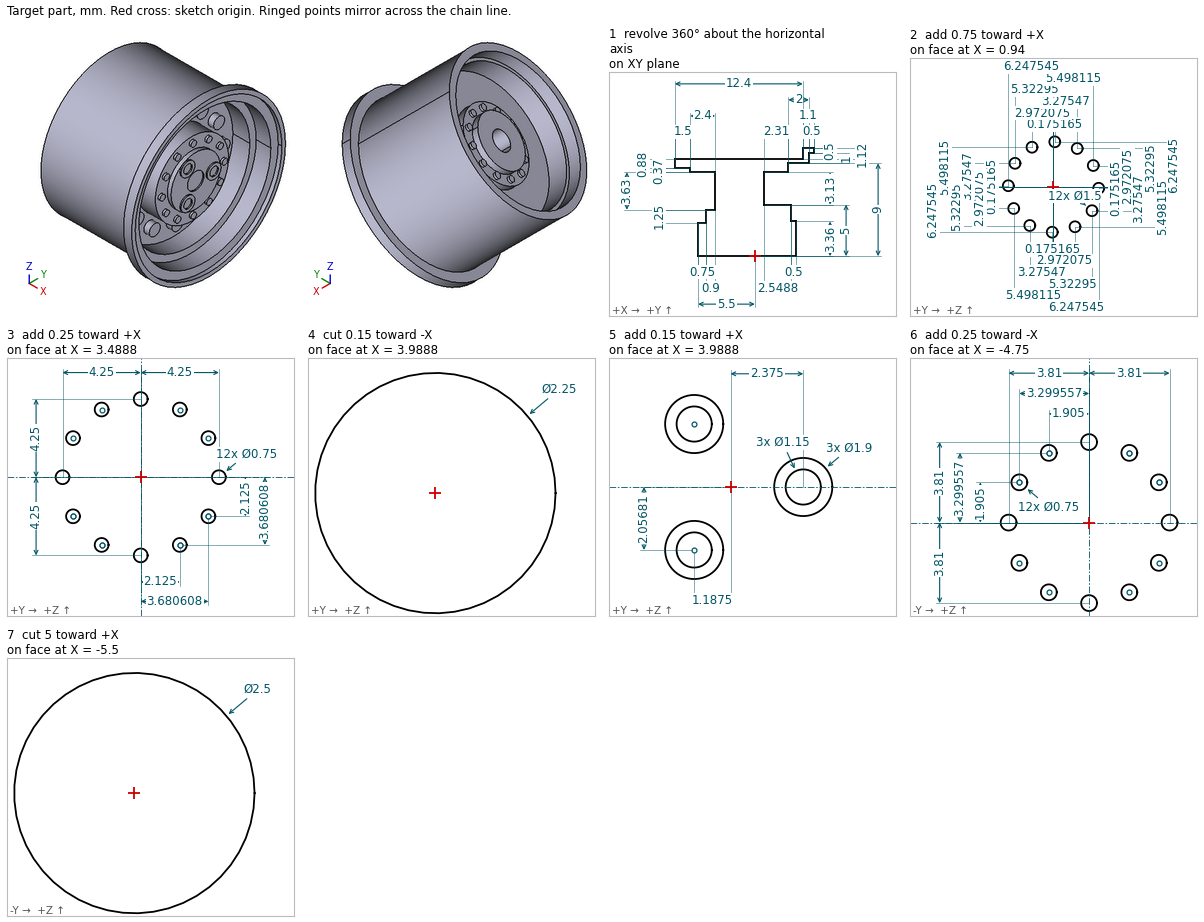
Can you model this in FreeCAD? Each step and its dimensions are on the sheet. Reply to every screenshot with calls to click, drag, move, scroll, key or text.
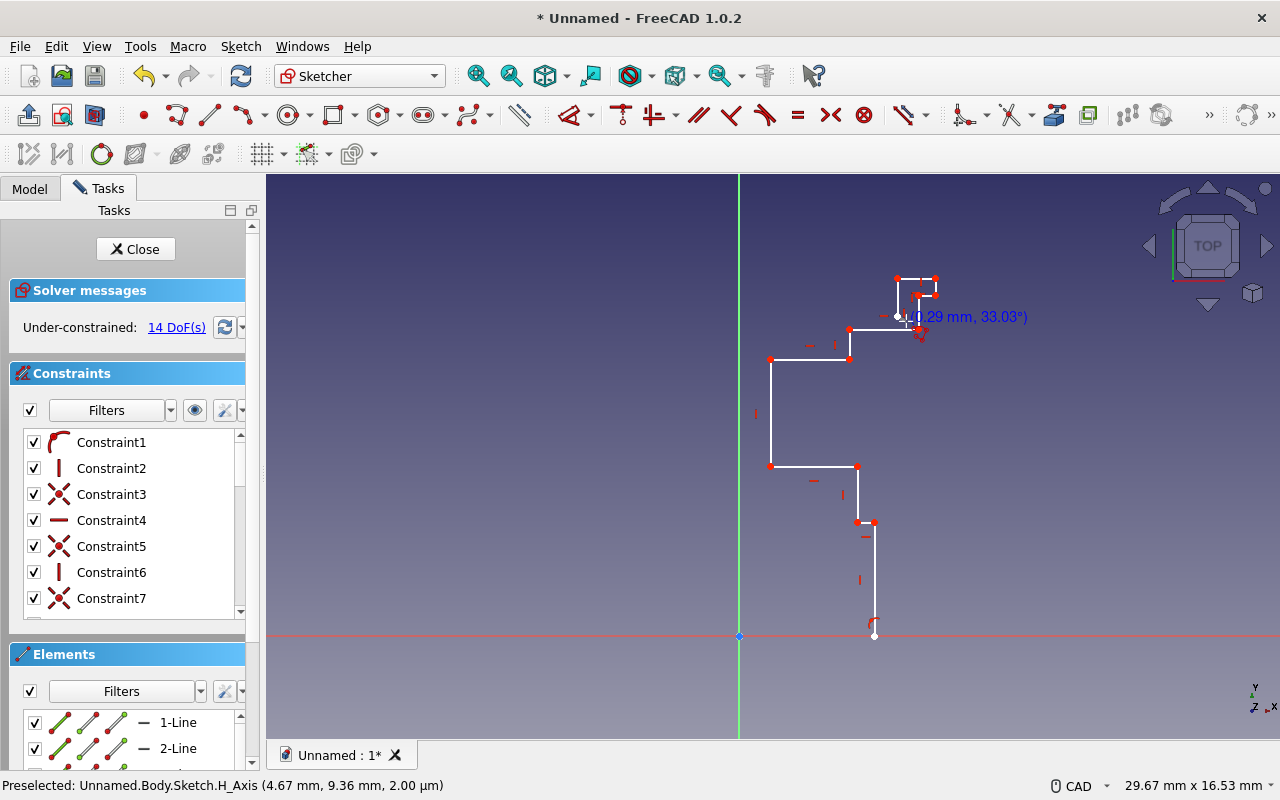
click(474, 316)
click(474, 346)
click(525, 346)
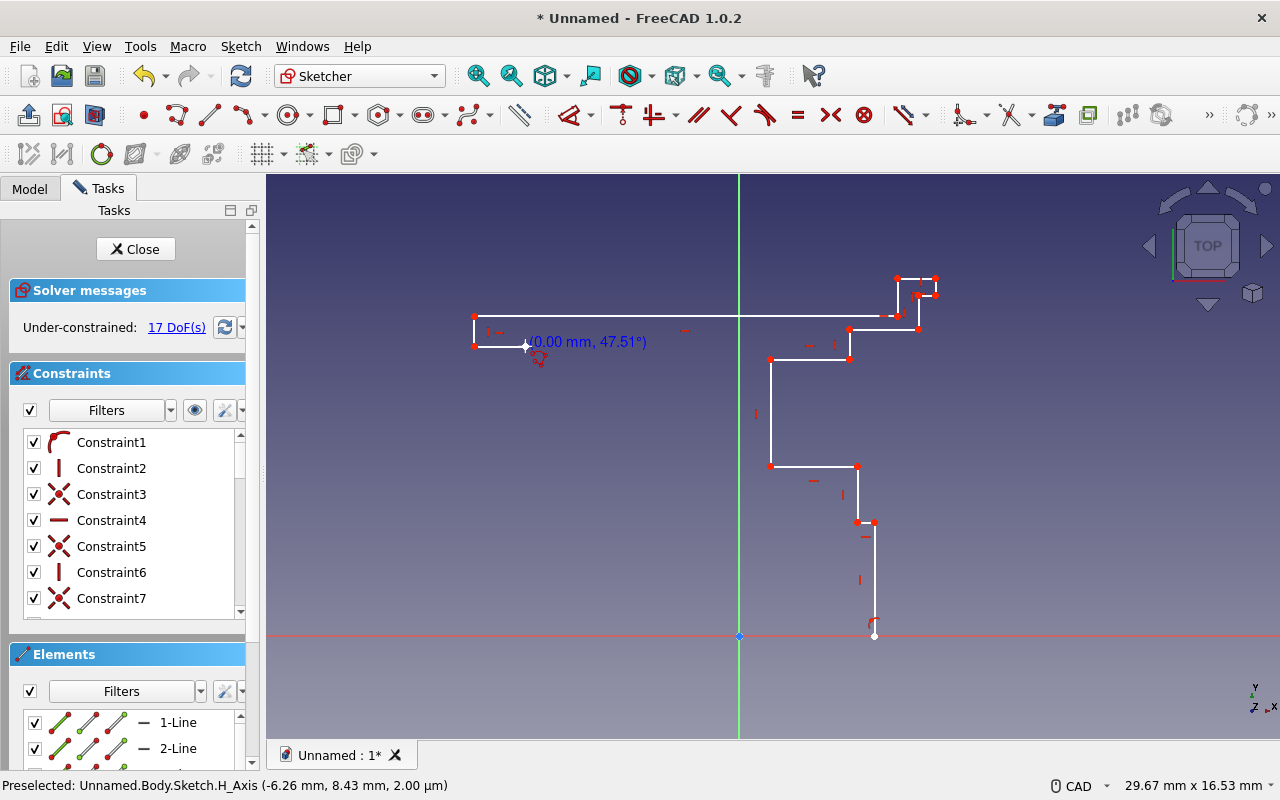
scroll(525, 358, up, 2)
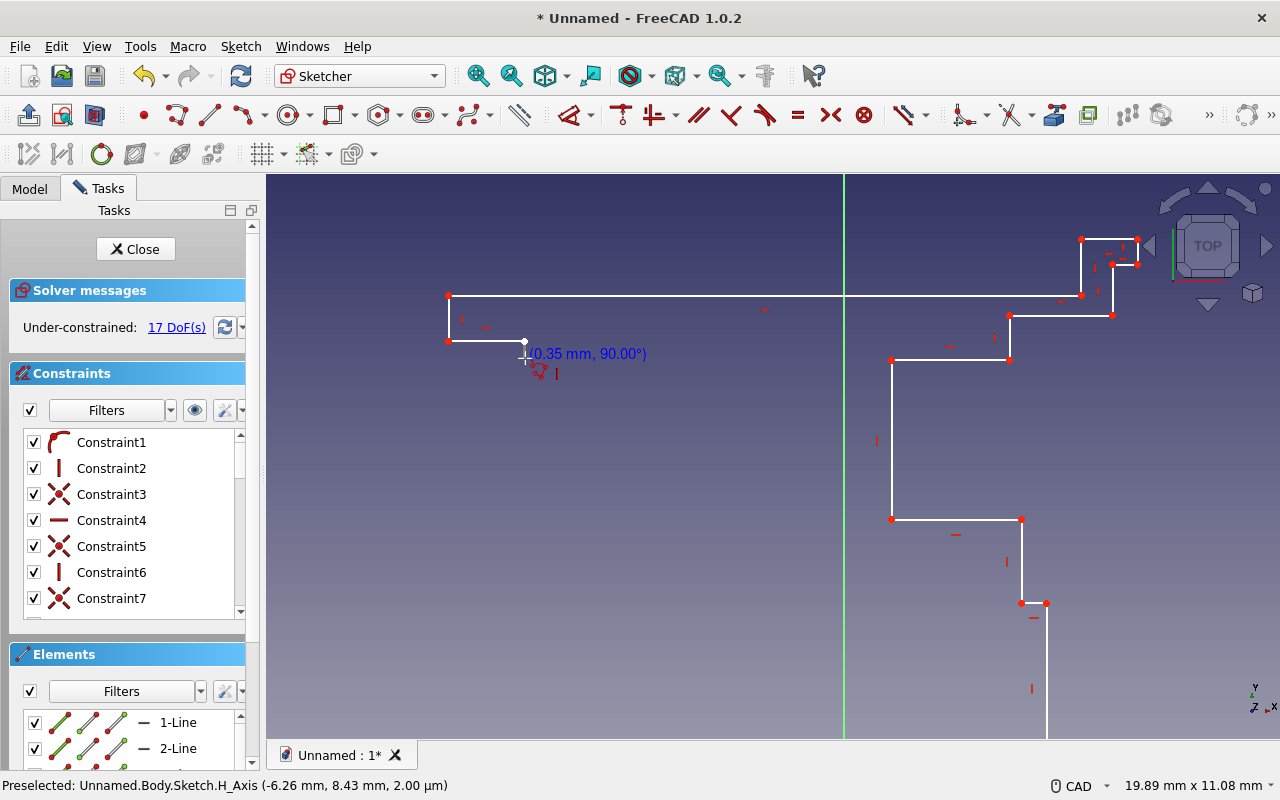
click(525, 358)
click(648, 358)
click(648, 543)
click(602, 543)
click(602, 607)
click(564, 607)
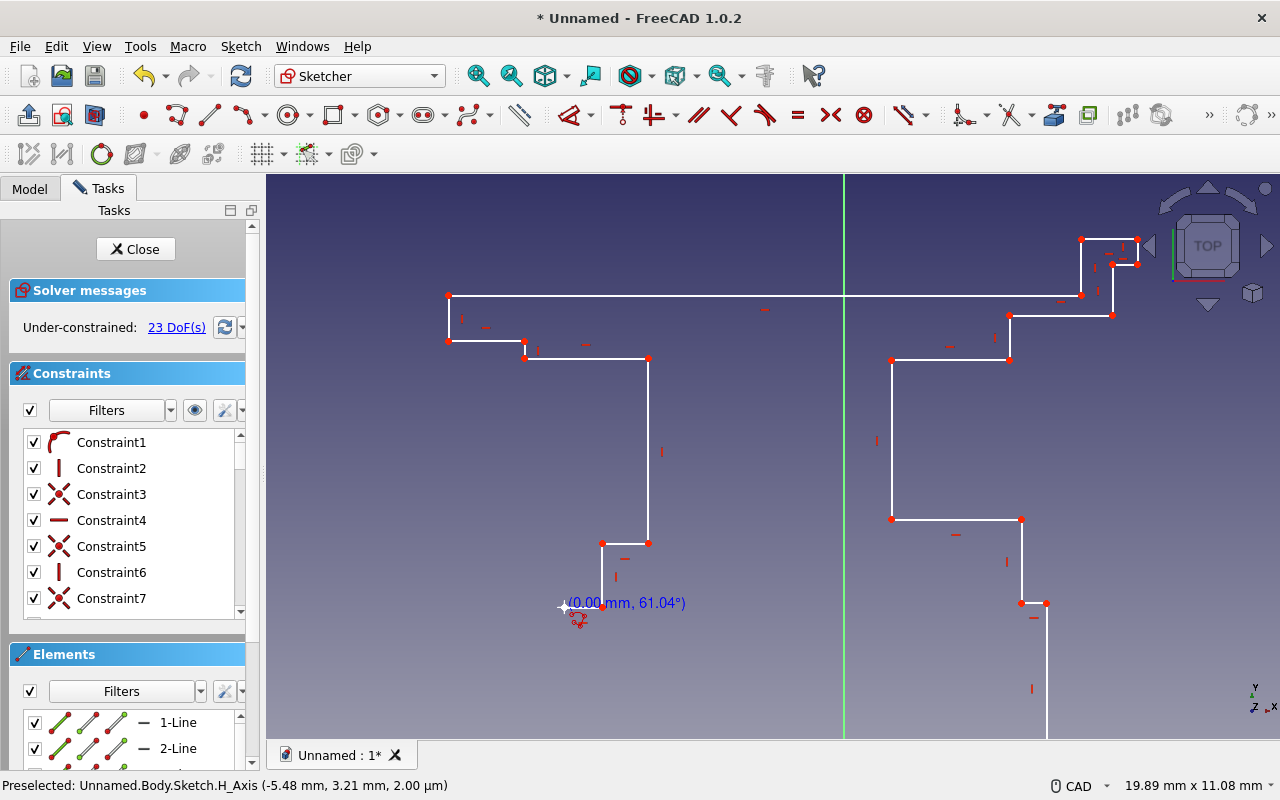
scroll(524, 358, down, 2)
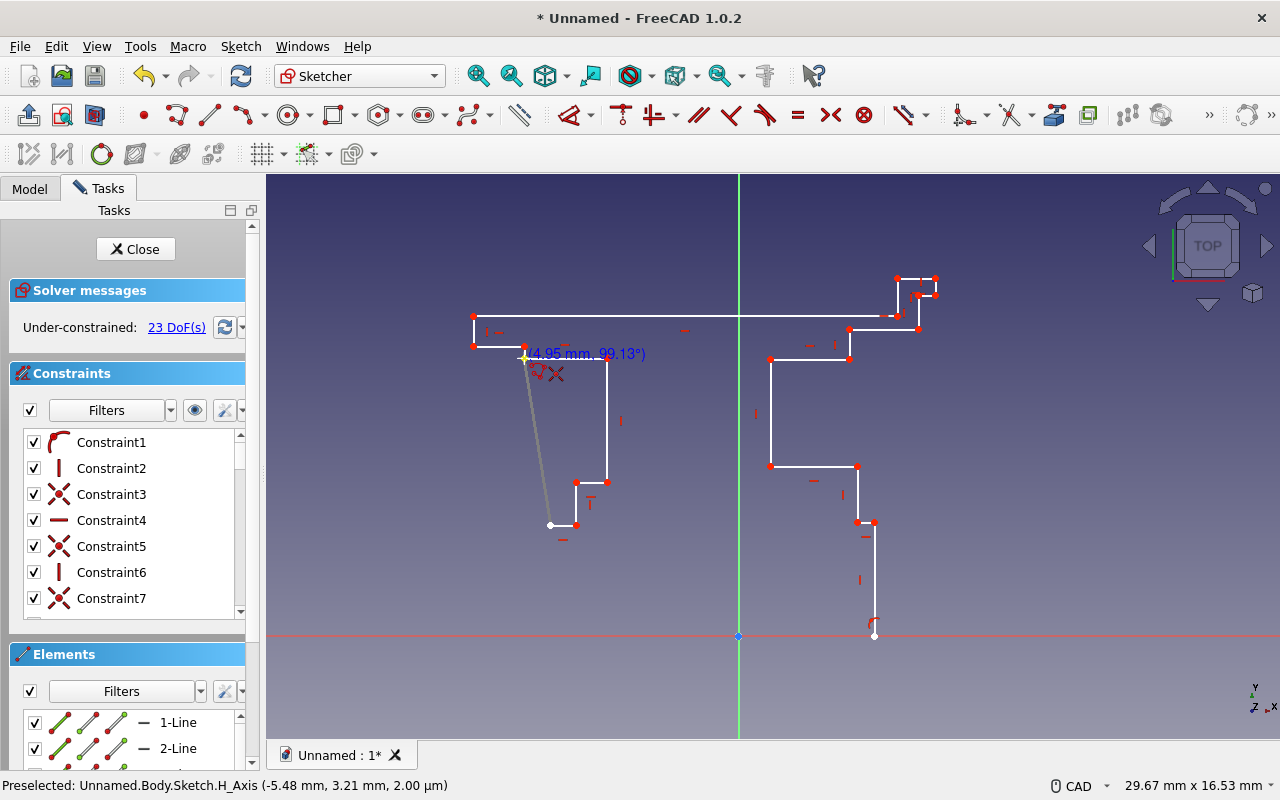
click(551, 627)
click(875, 636)
key(Escape)
key(Escape)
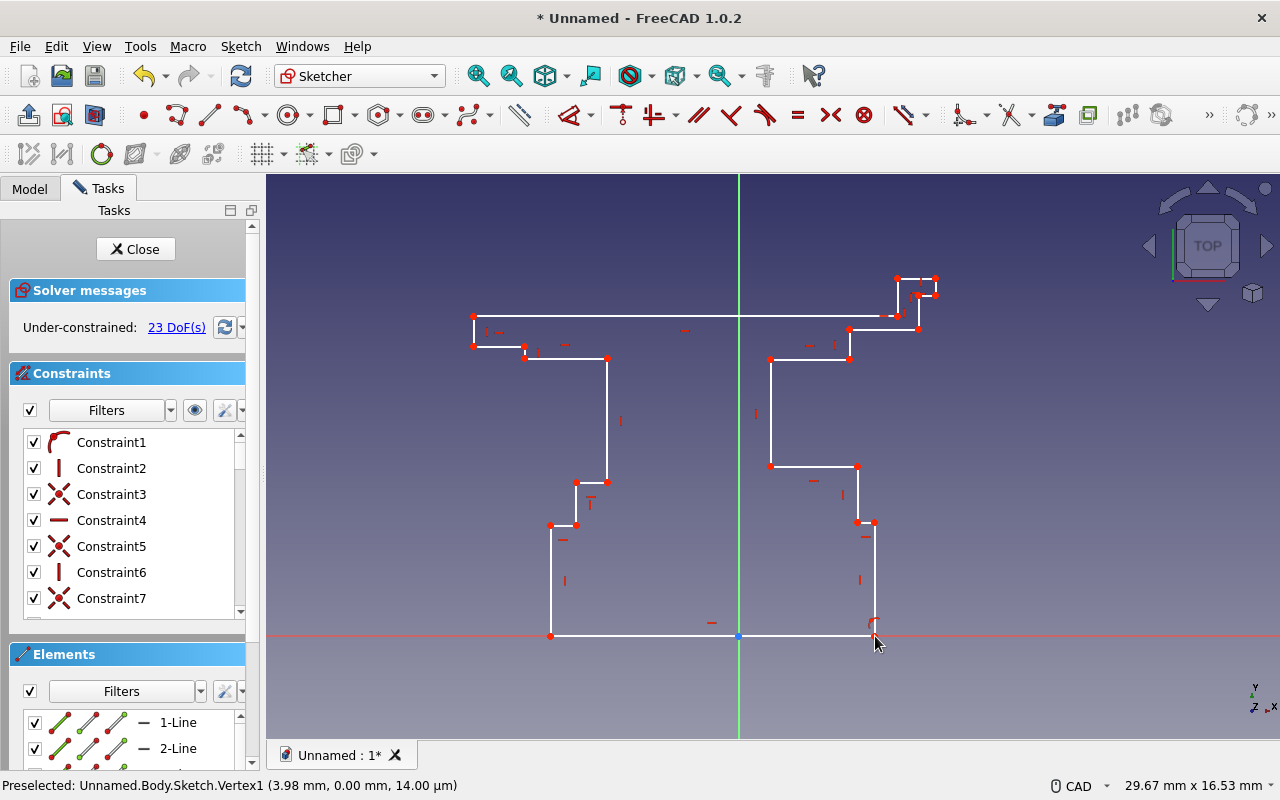
click(568, 116)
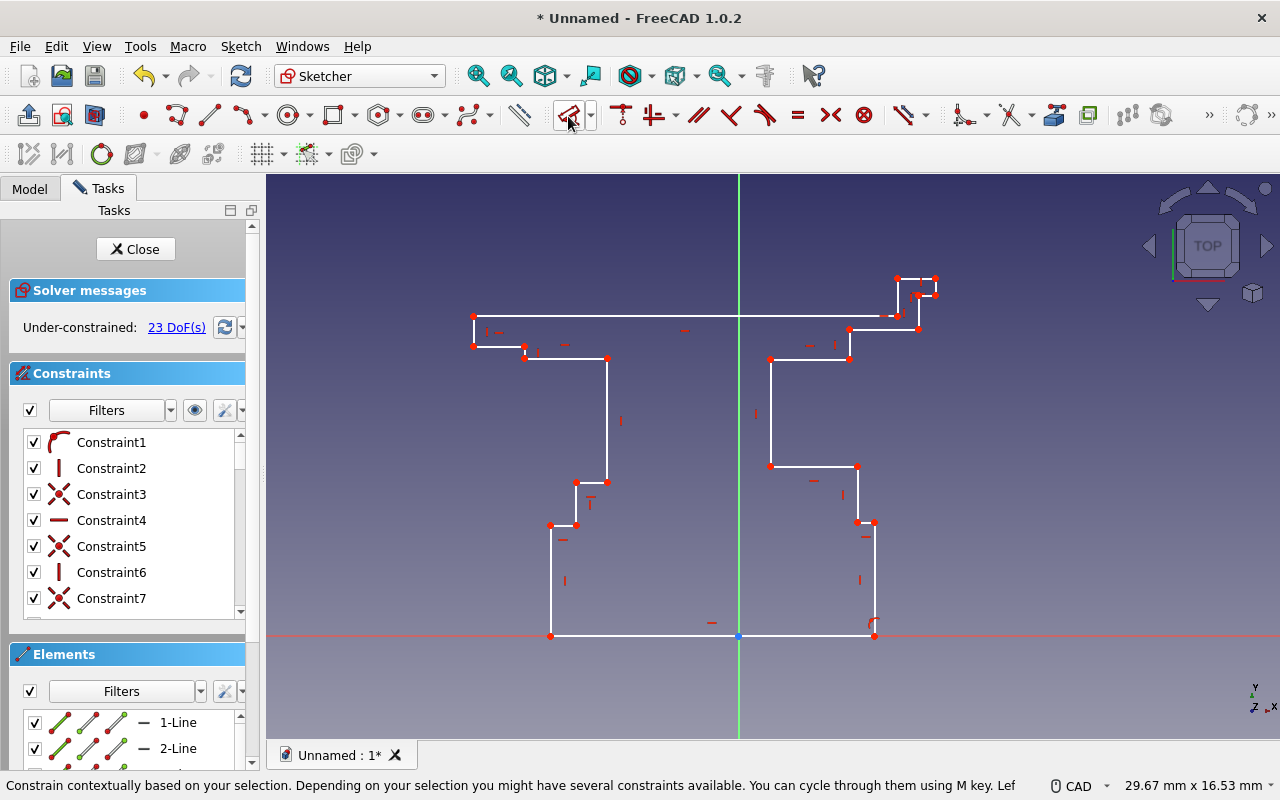
click(870, 330)
click(884, 296)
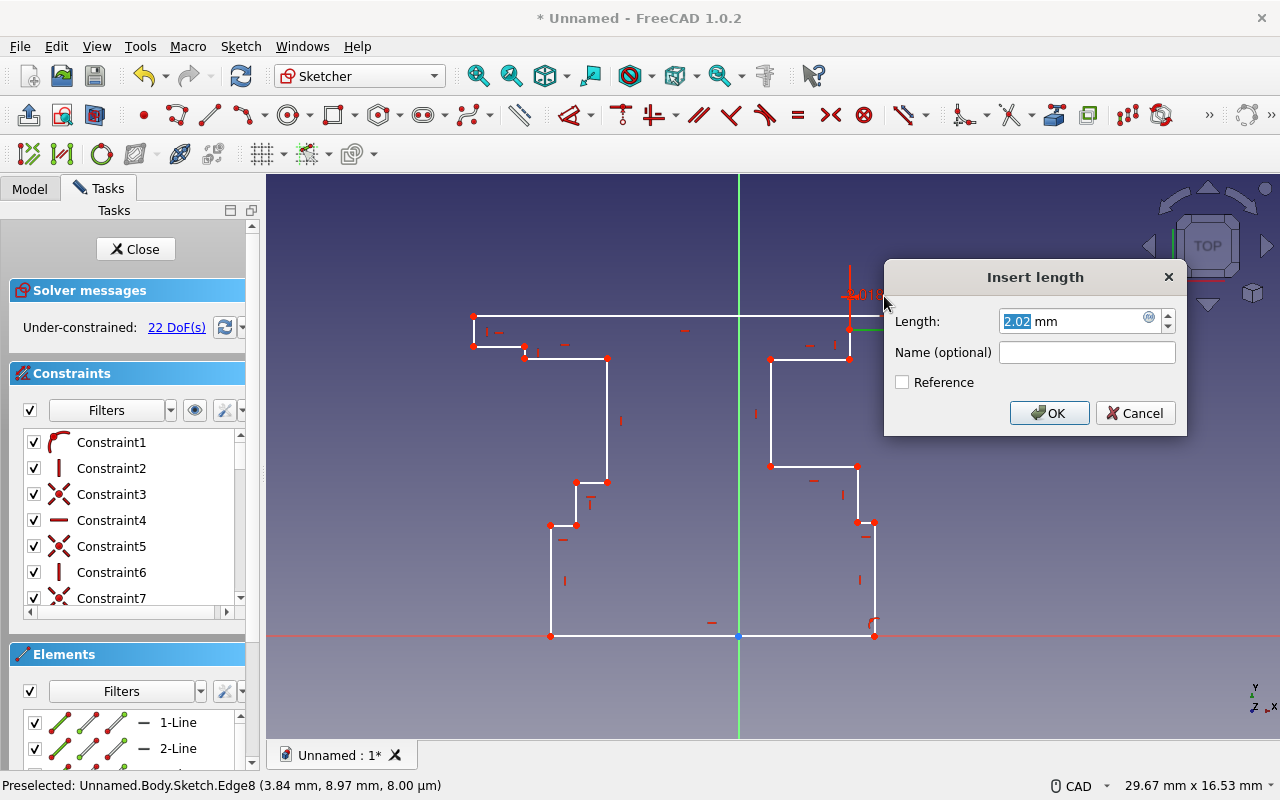
text(2)
key(Return)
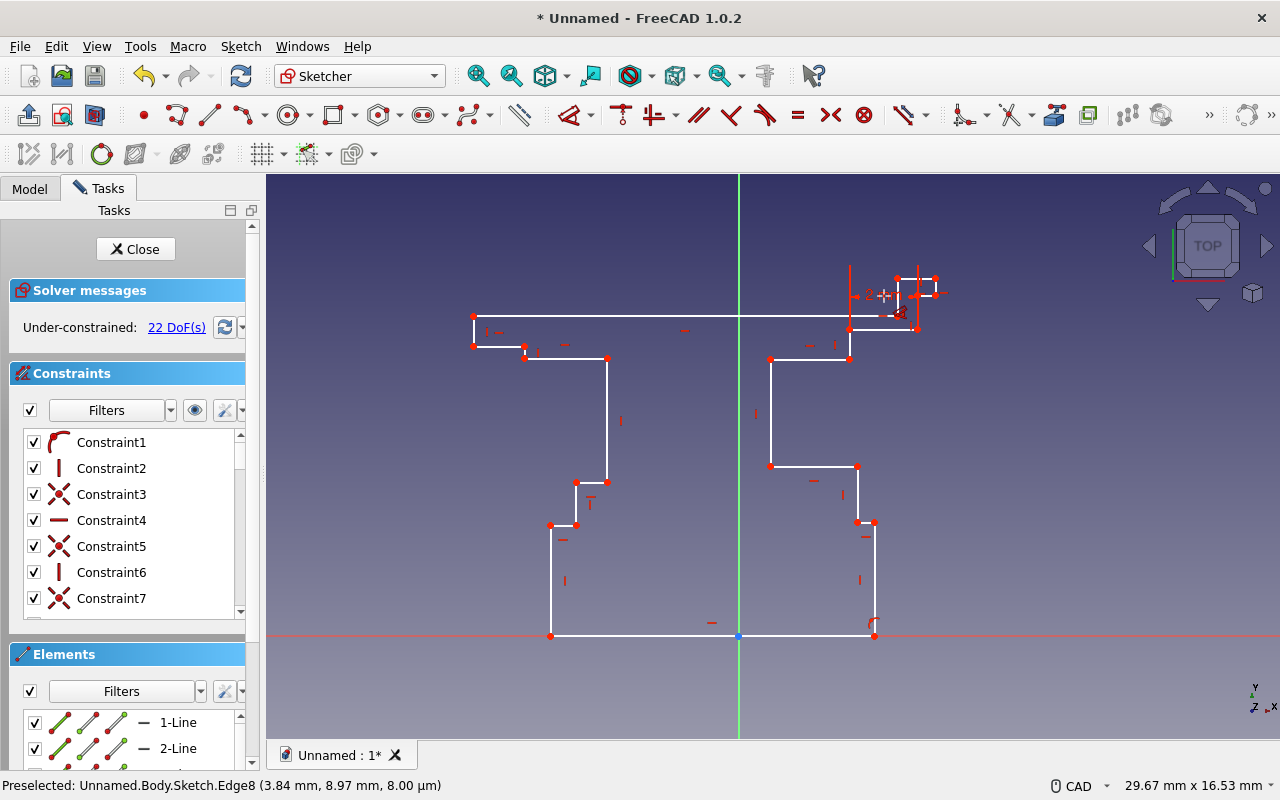
scroll(918, 319, up, 2)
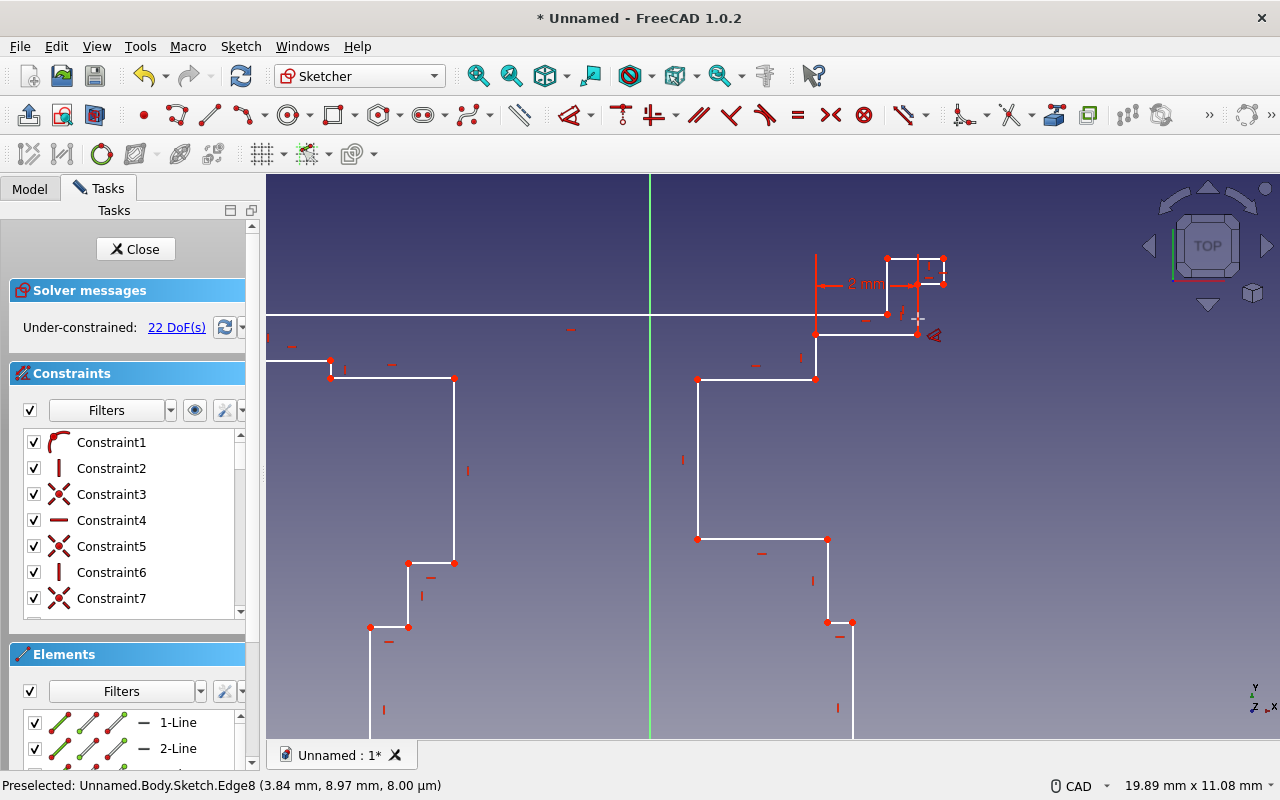
click(918, 320)
click(952, 309)